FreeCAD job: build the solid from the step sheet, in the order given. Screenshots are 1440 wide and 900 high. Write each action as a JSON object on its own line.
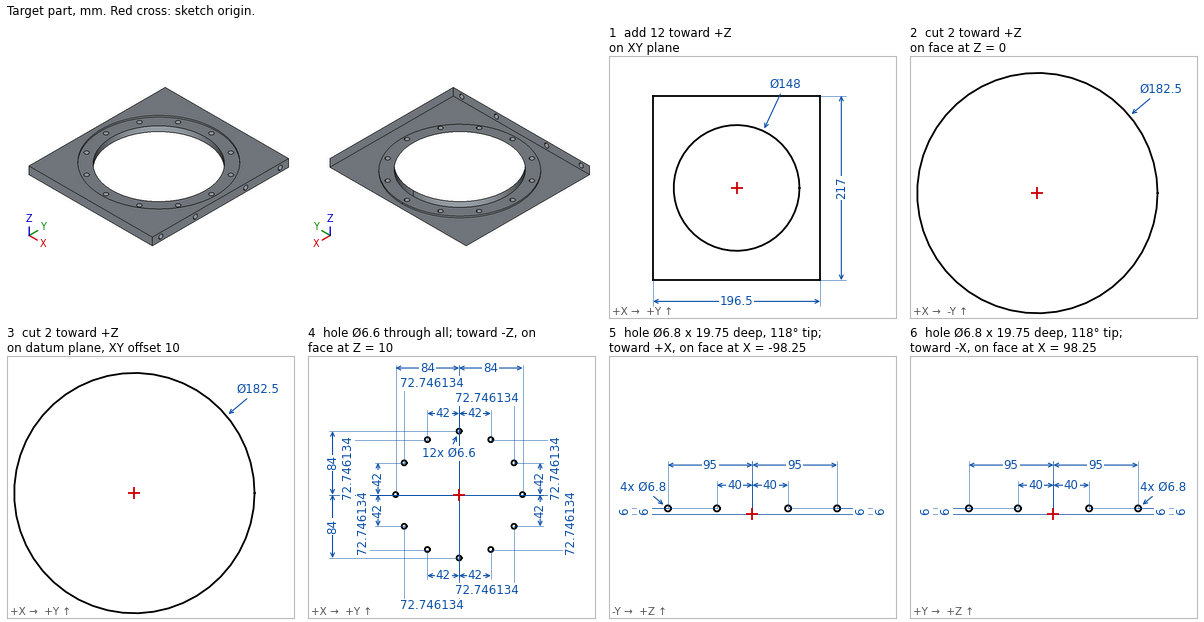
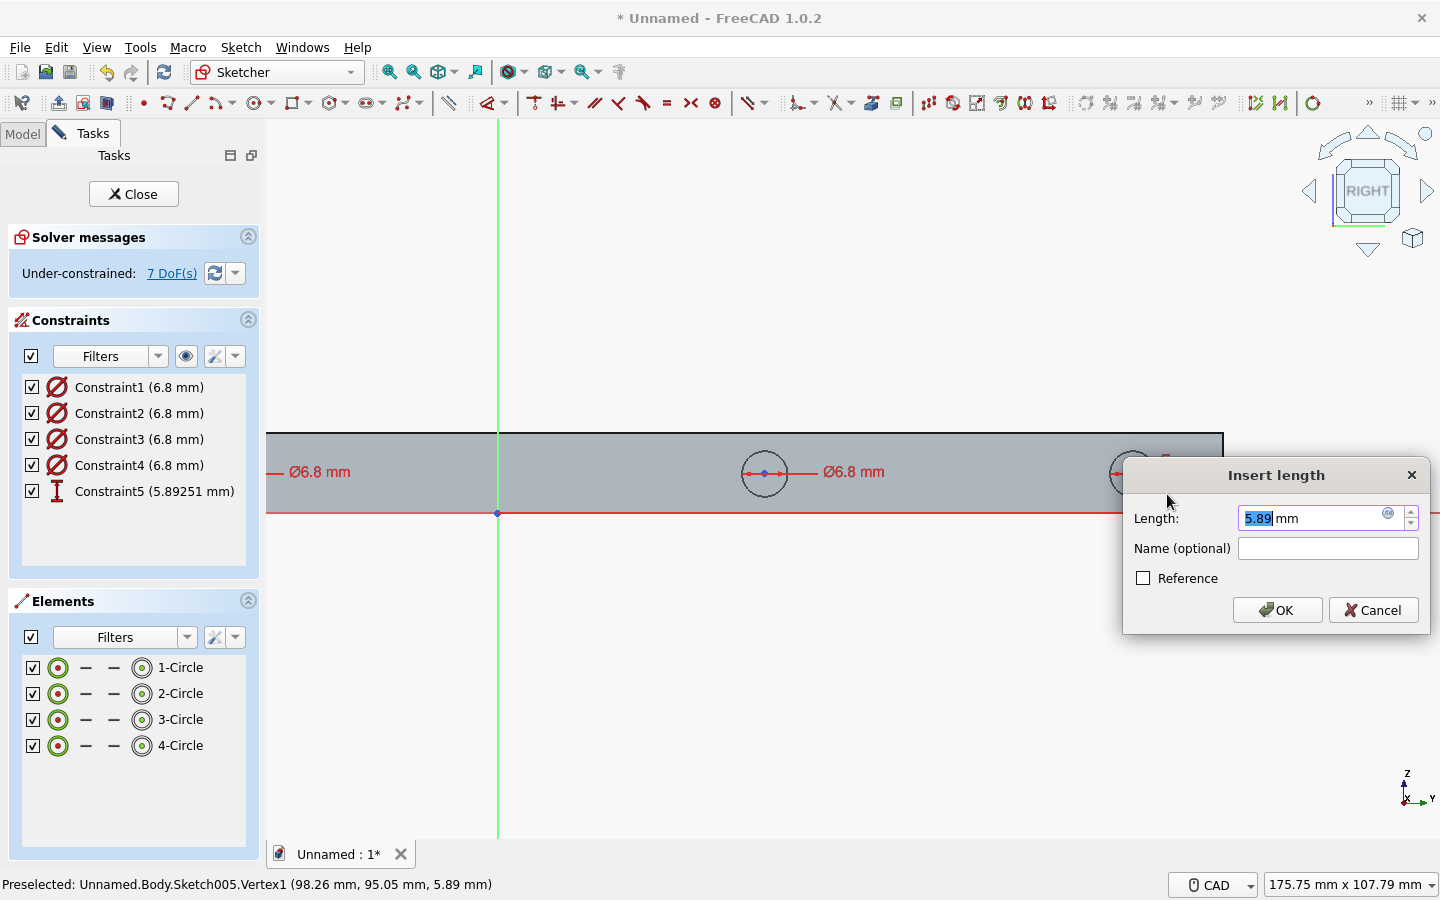
{"action": "type", "text": "6"}
{"action": "key", "text": "Return"}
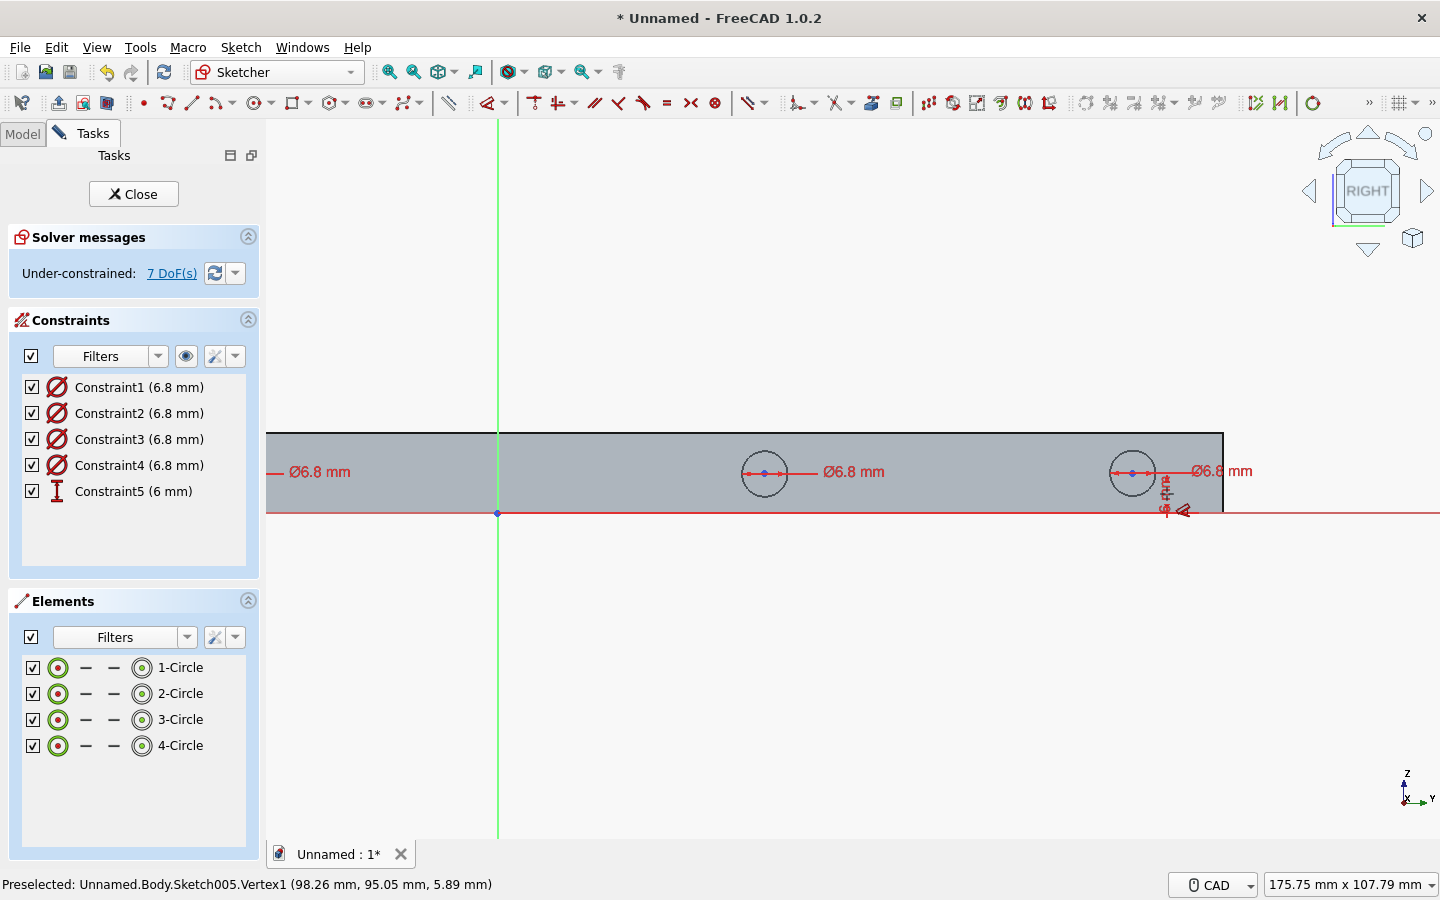
{"action": "left_click", "coordinate": [765, 474]}
{"action": "left_click", "coordinate": [799, 494]}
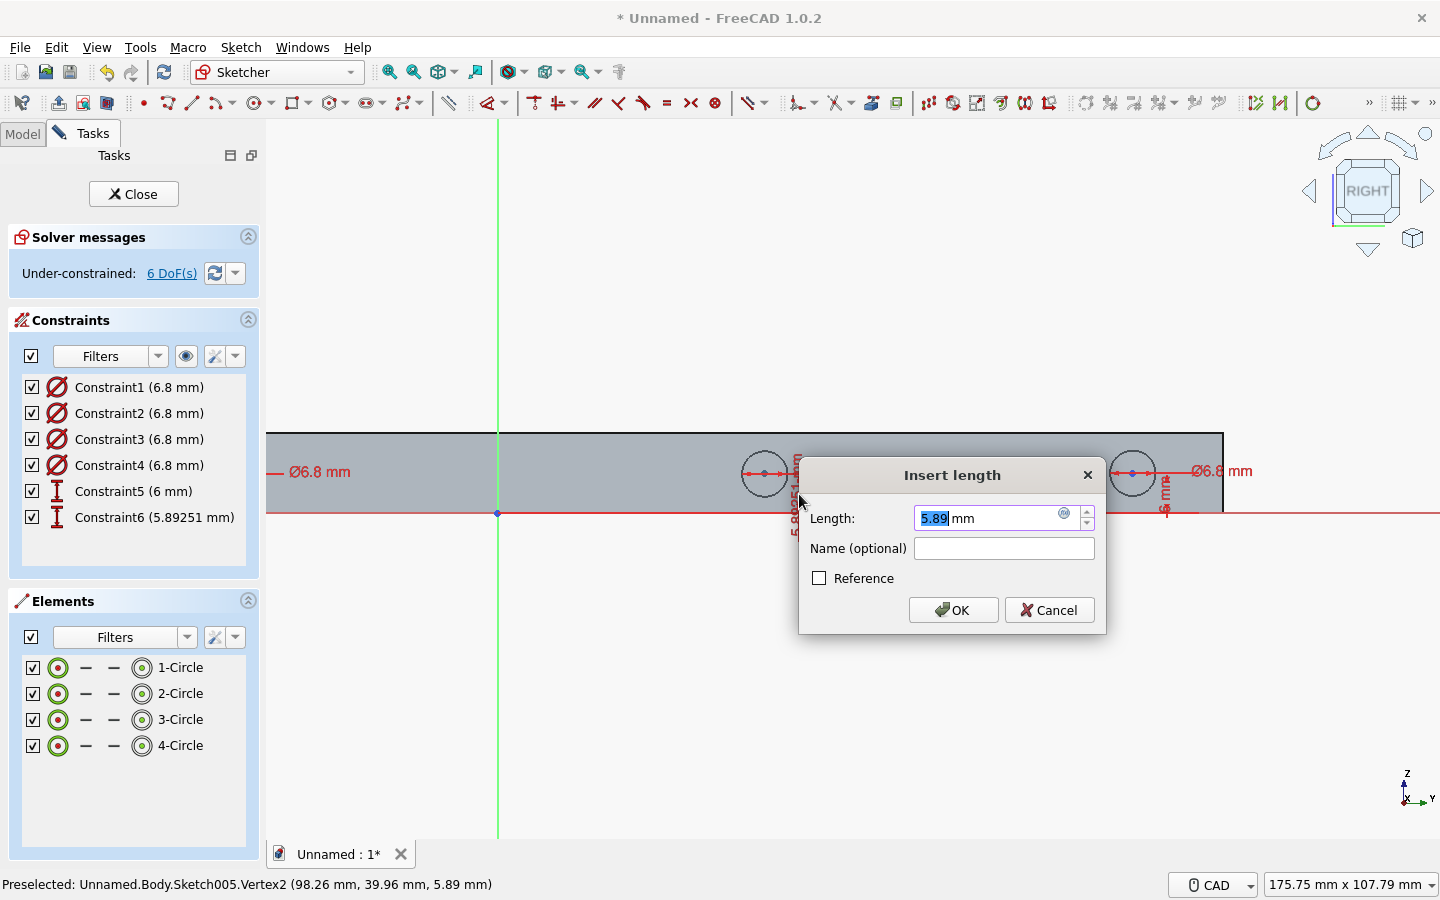
{"action": "type", "text": "6"}
{"action": "key", "text": "Return"}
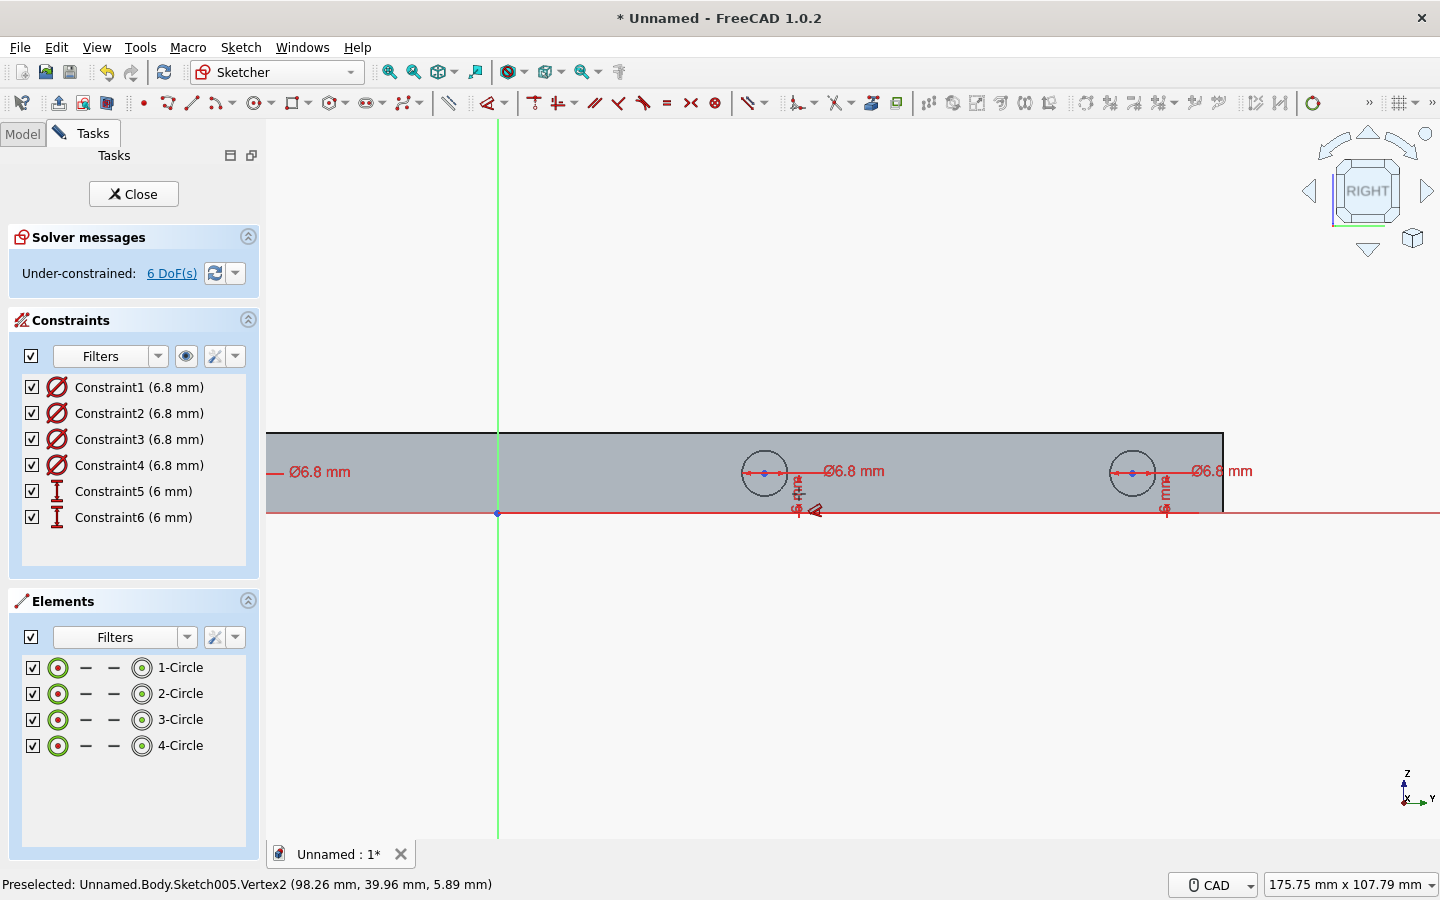
{"action": "scroll", "coordinate": [1133, 475], "scroll_direction": "down", "scroll_amount": 3}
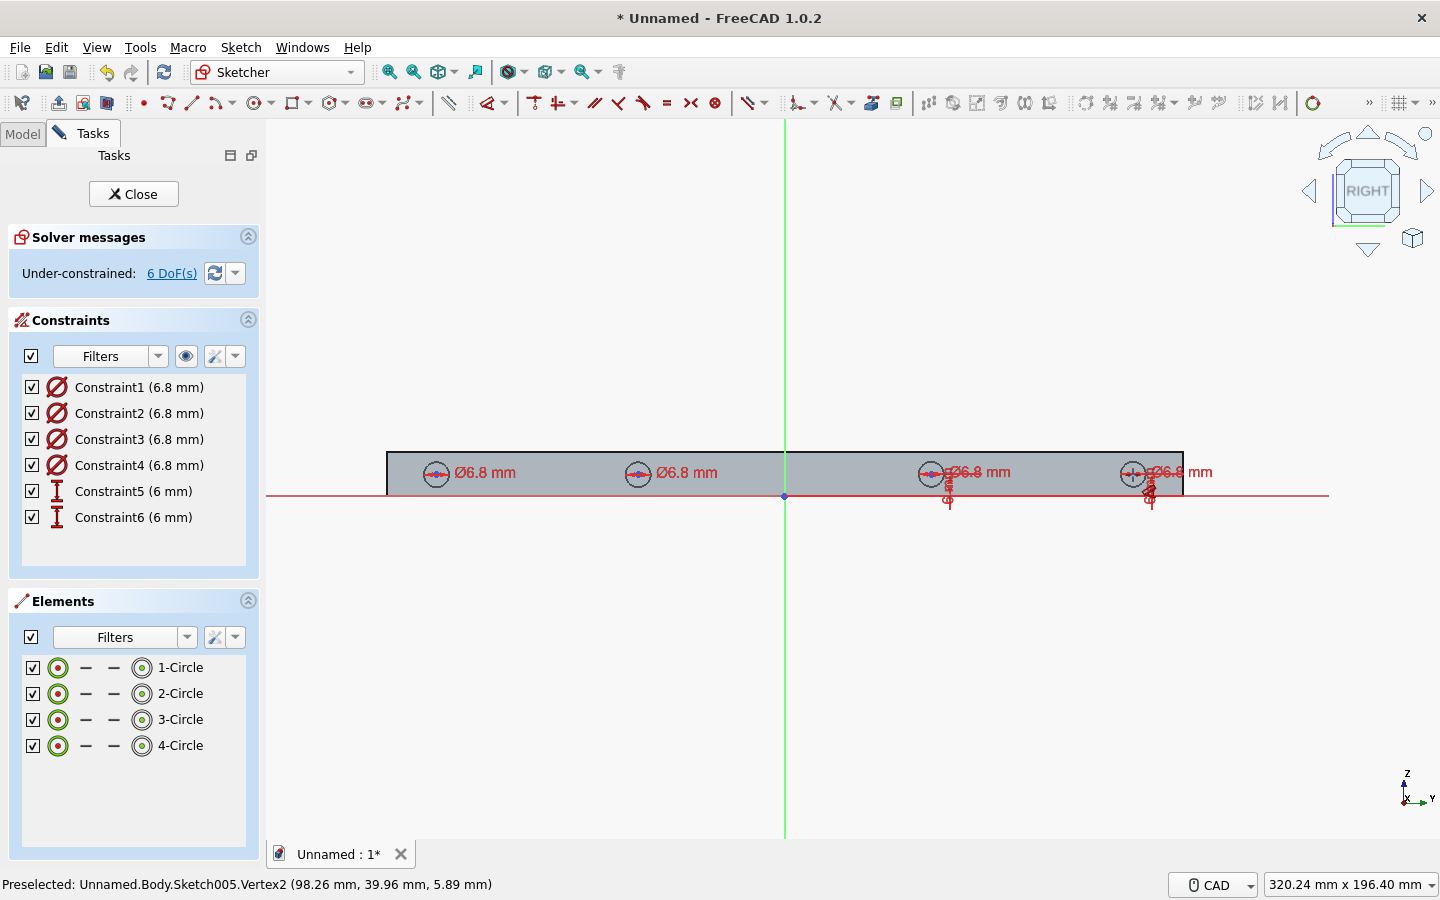
{"action": "scroll", "coordinate": [638, 475], "scroll_direction": "up", "scroll_amount": 3}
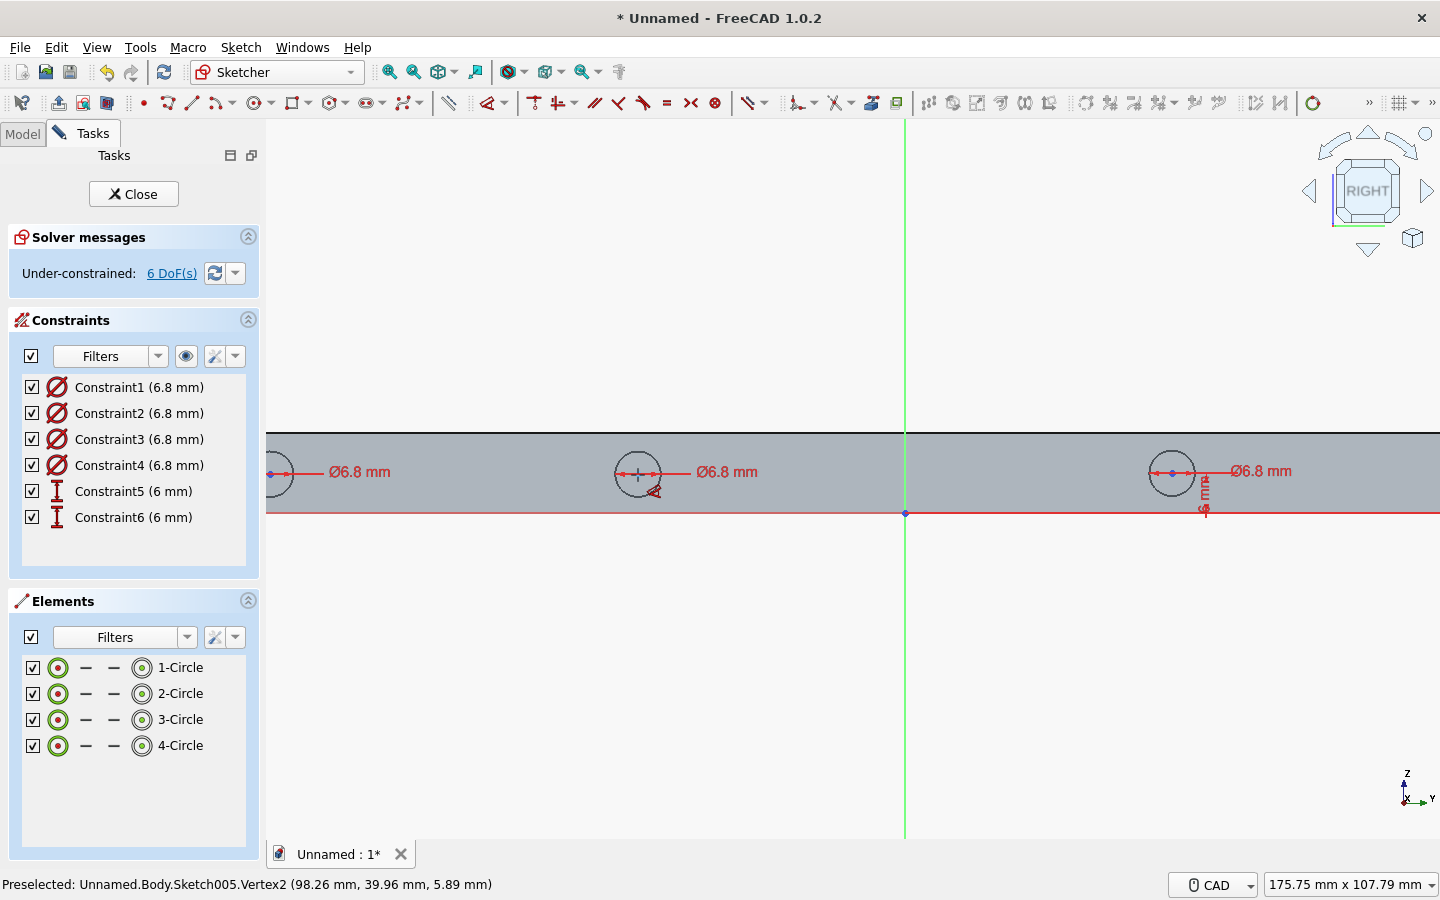
{"action": "left_click", "coordinate": [638, 474]}
{"action": "left_click", "coordinate": [604, 494]}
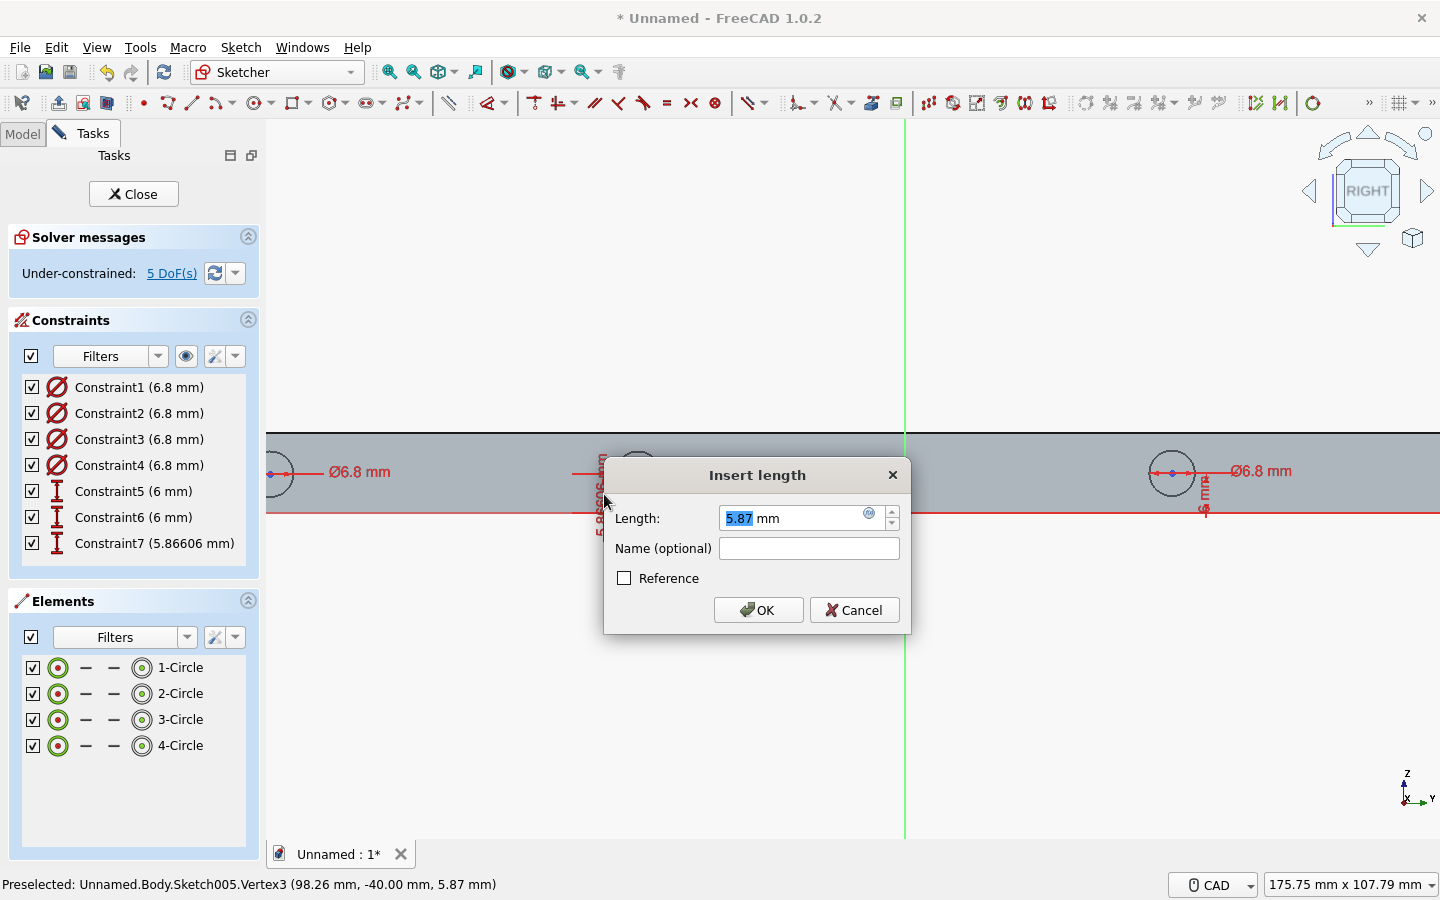
{"action": "type", "text": "6"}
{"action": "key", "text": "Return"}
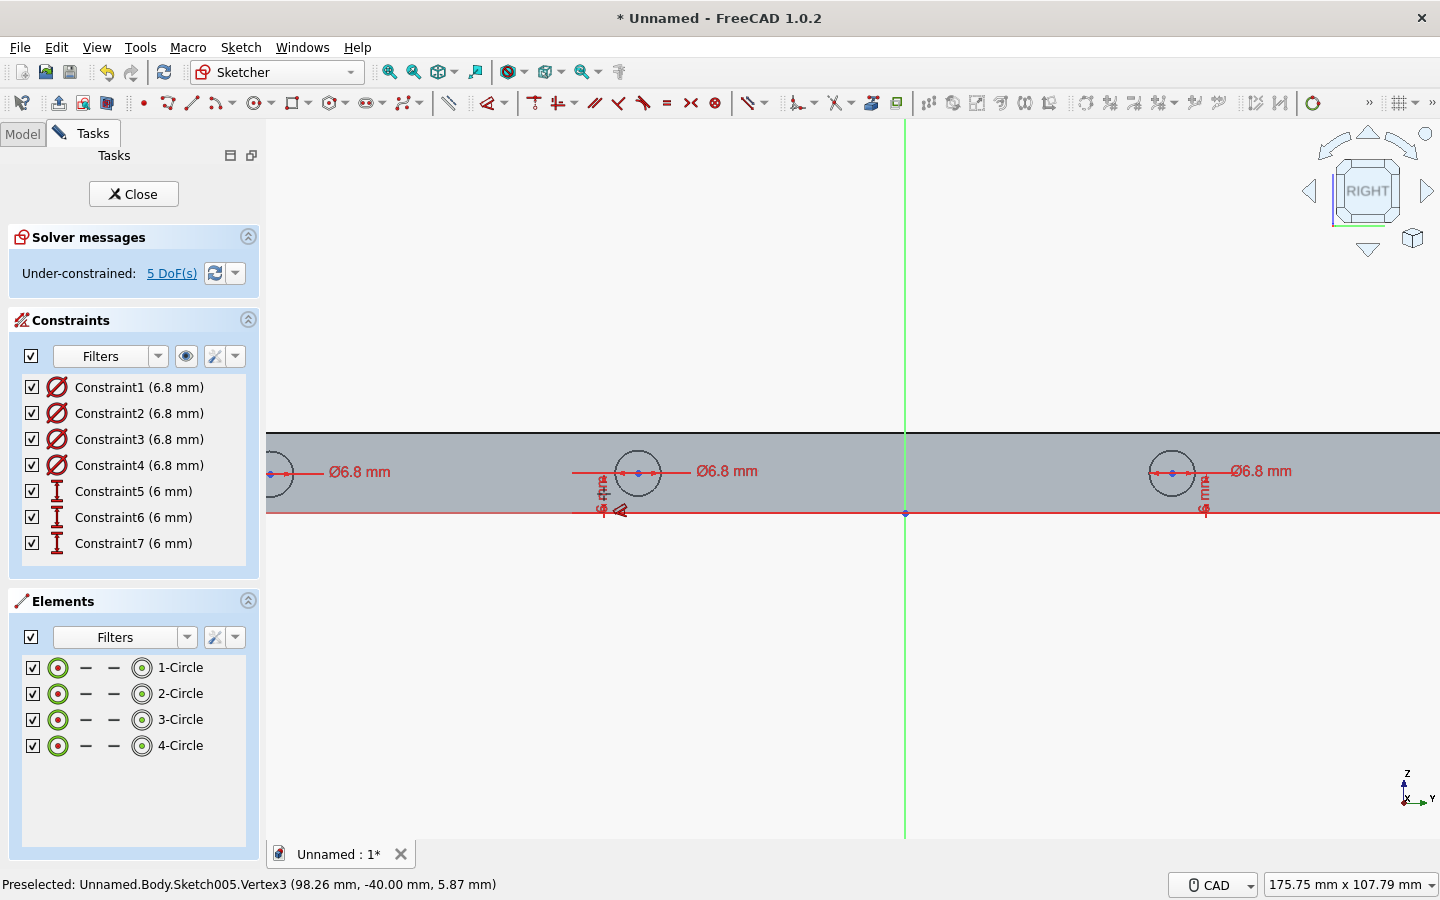
{"action": "scroll", "coordinate": [638, 475], "scroll_direction": "down", "scroll_amount": 3}